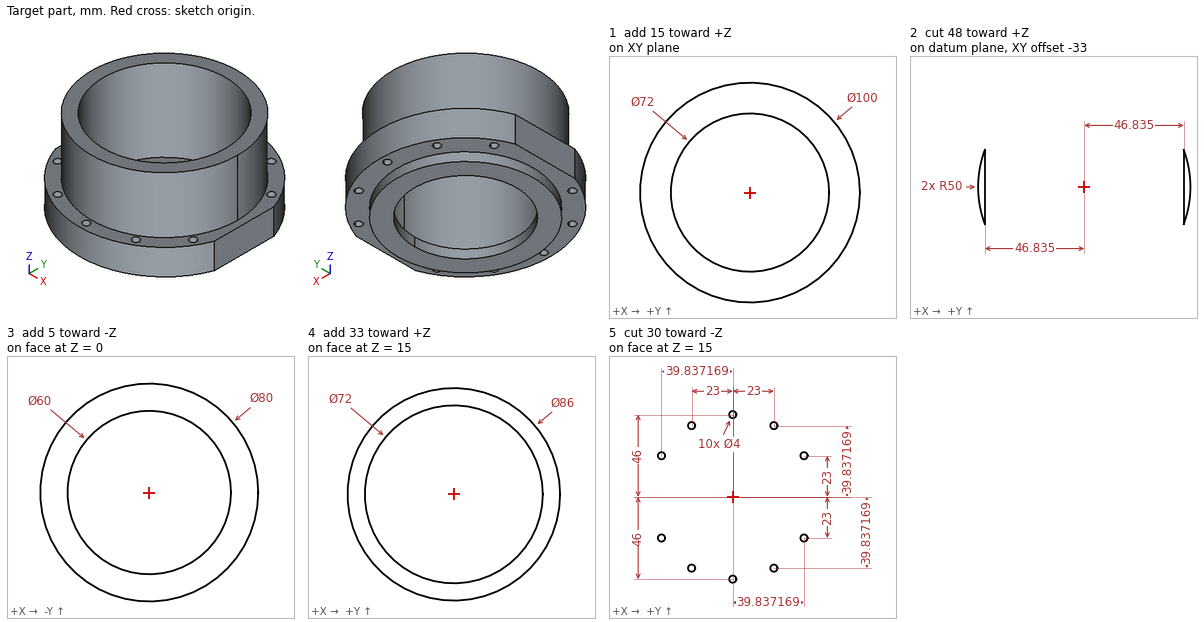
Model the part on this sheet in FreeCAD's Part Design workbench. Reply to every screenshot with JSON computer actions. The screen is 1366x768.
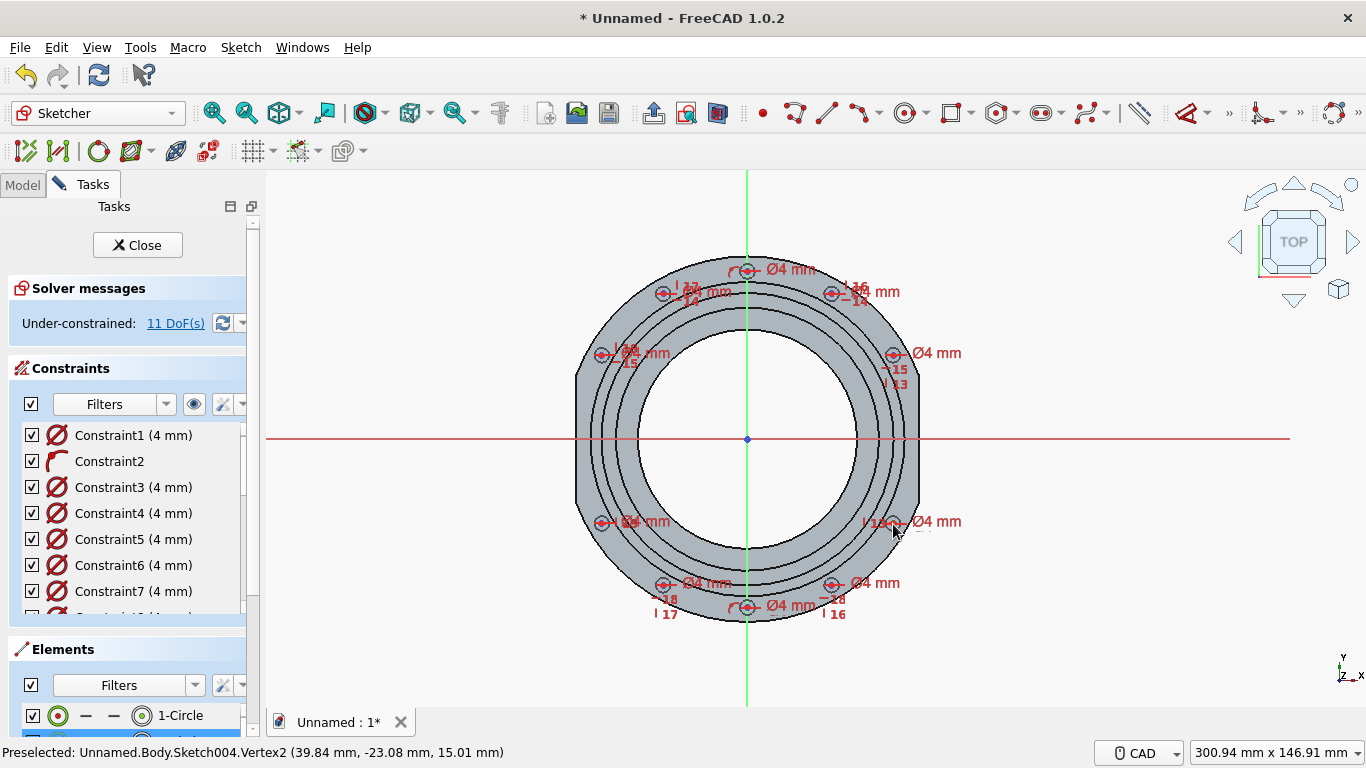
{"action": "left_click", "coordinate": [602, 523]}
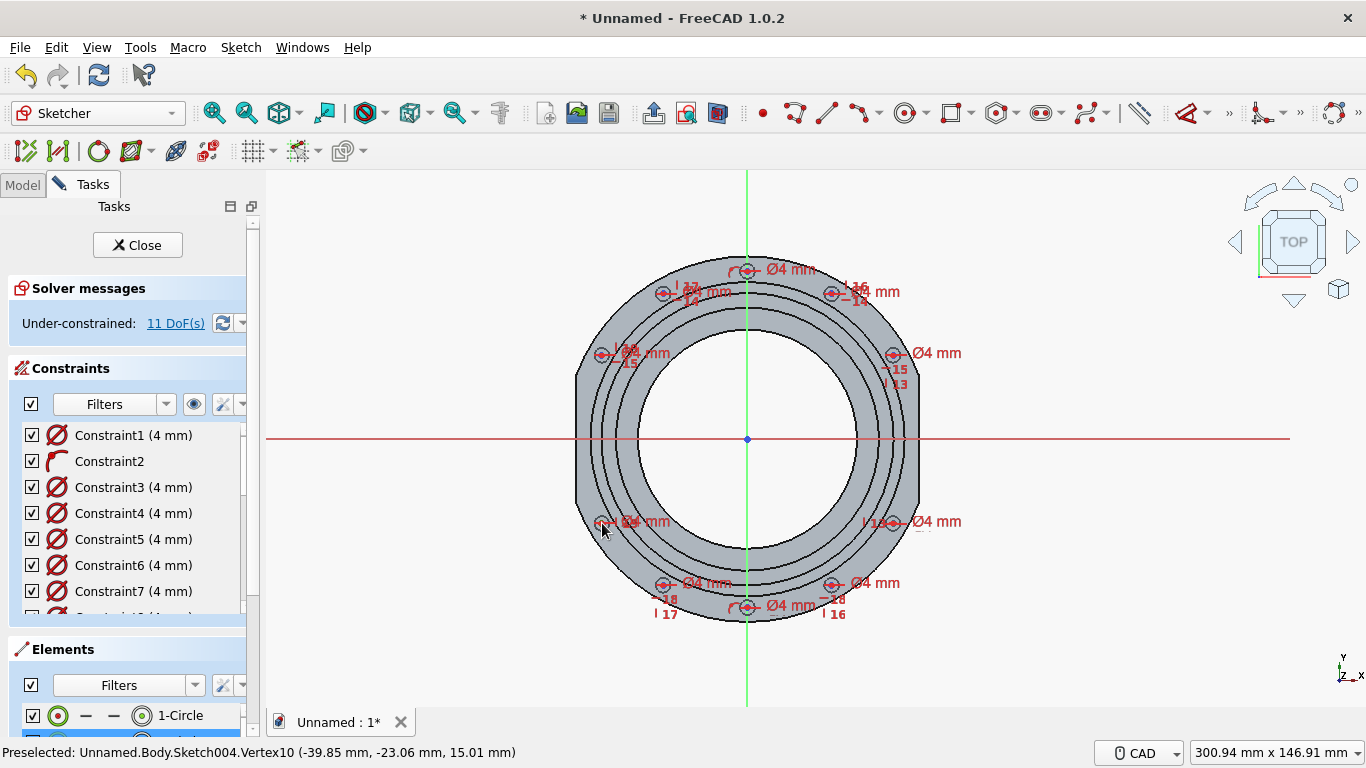
{"action": "key", "text": "h"}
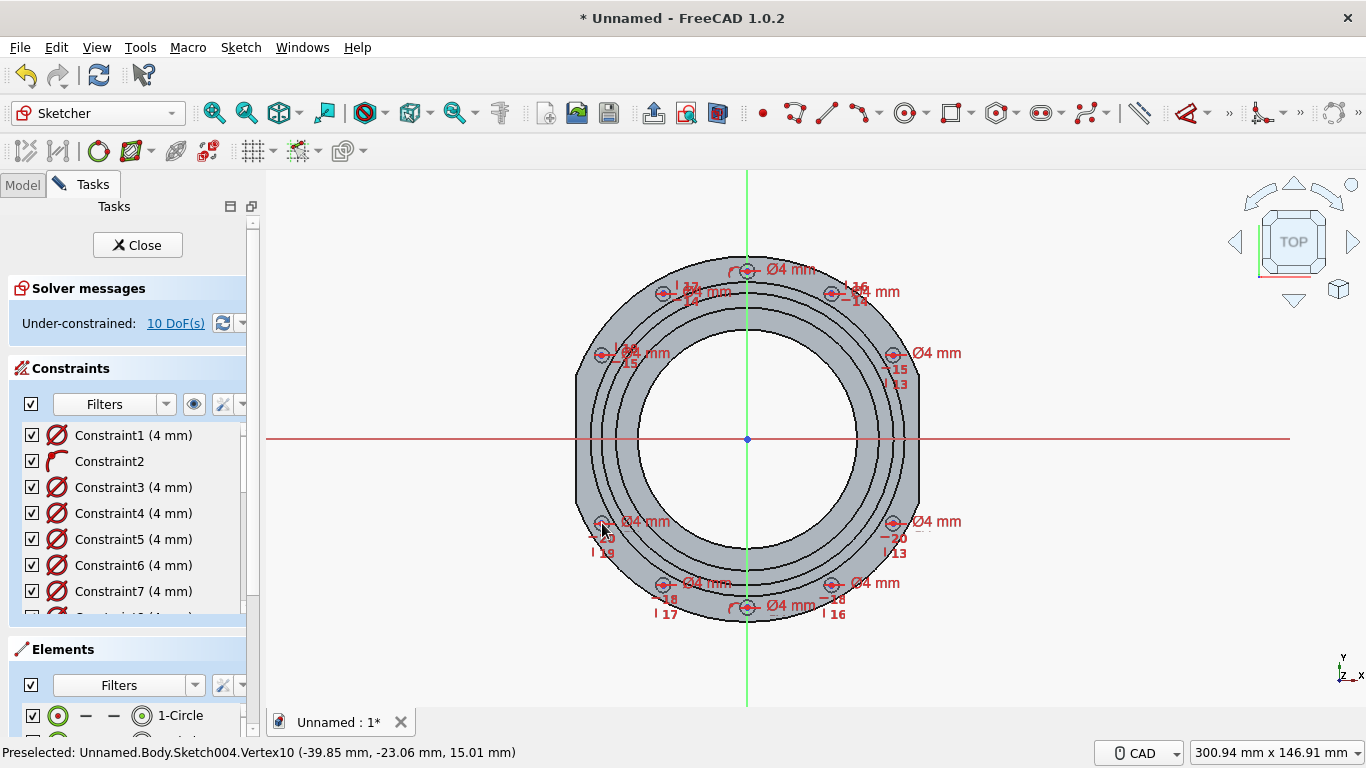
{"action": "left_click", "coordinate": [1186, 114]}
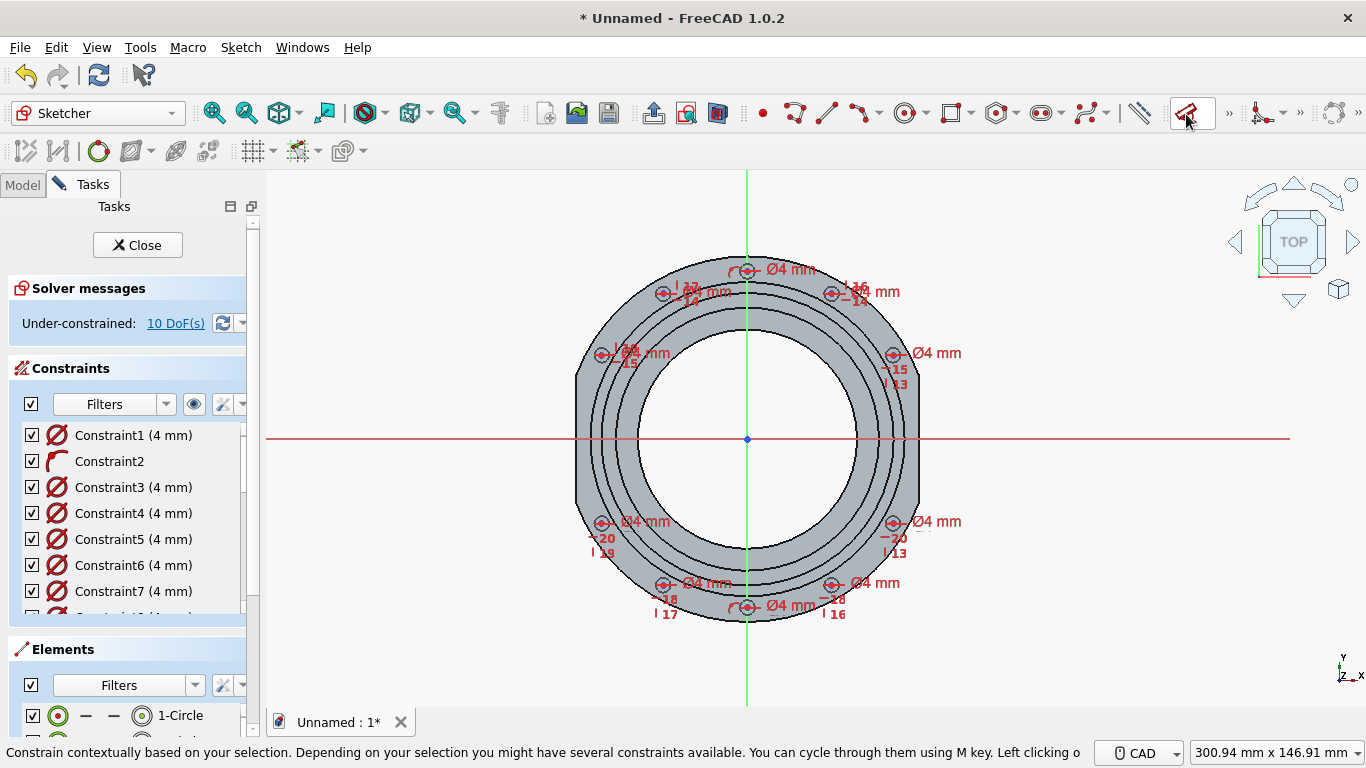
{"action": "left_click", "coordinate": [747, 271]}
{"action": "left_click", "coordinate": [781, 355]}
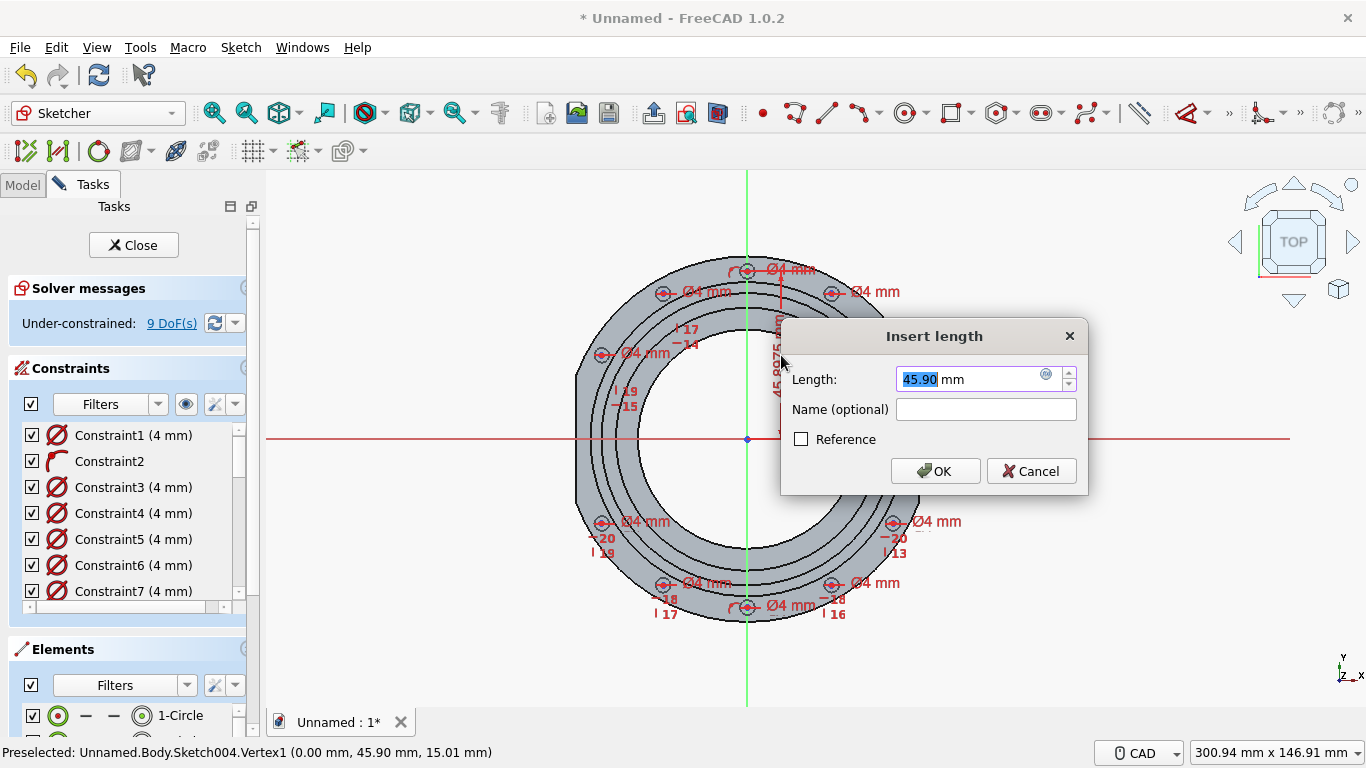
{"action": "type", "text": "46"}
{"action": "key", "text": "Return"}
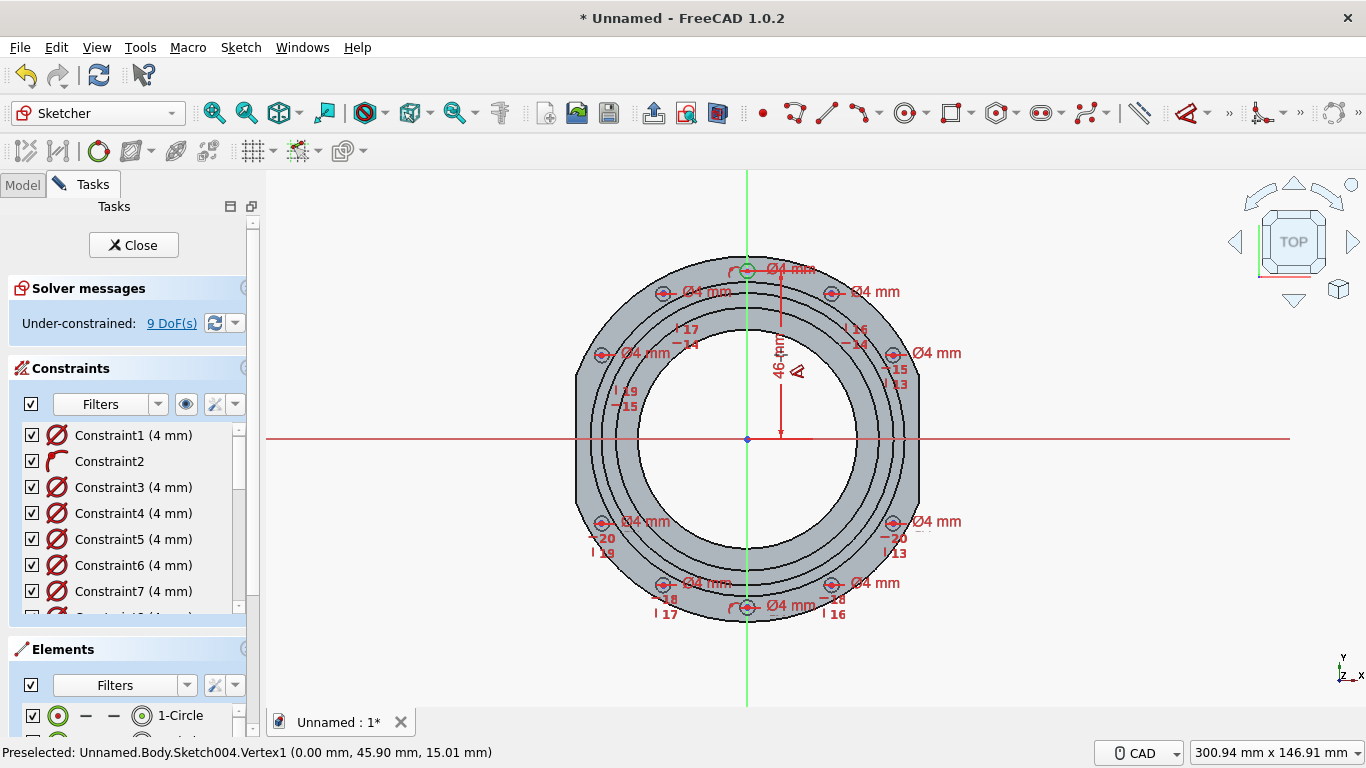
{"action": "left_click", "coordinate": [893, 524]}
{"action": "left_click", "coordinate": [927, 481]}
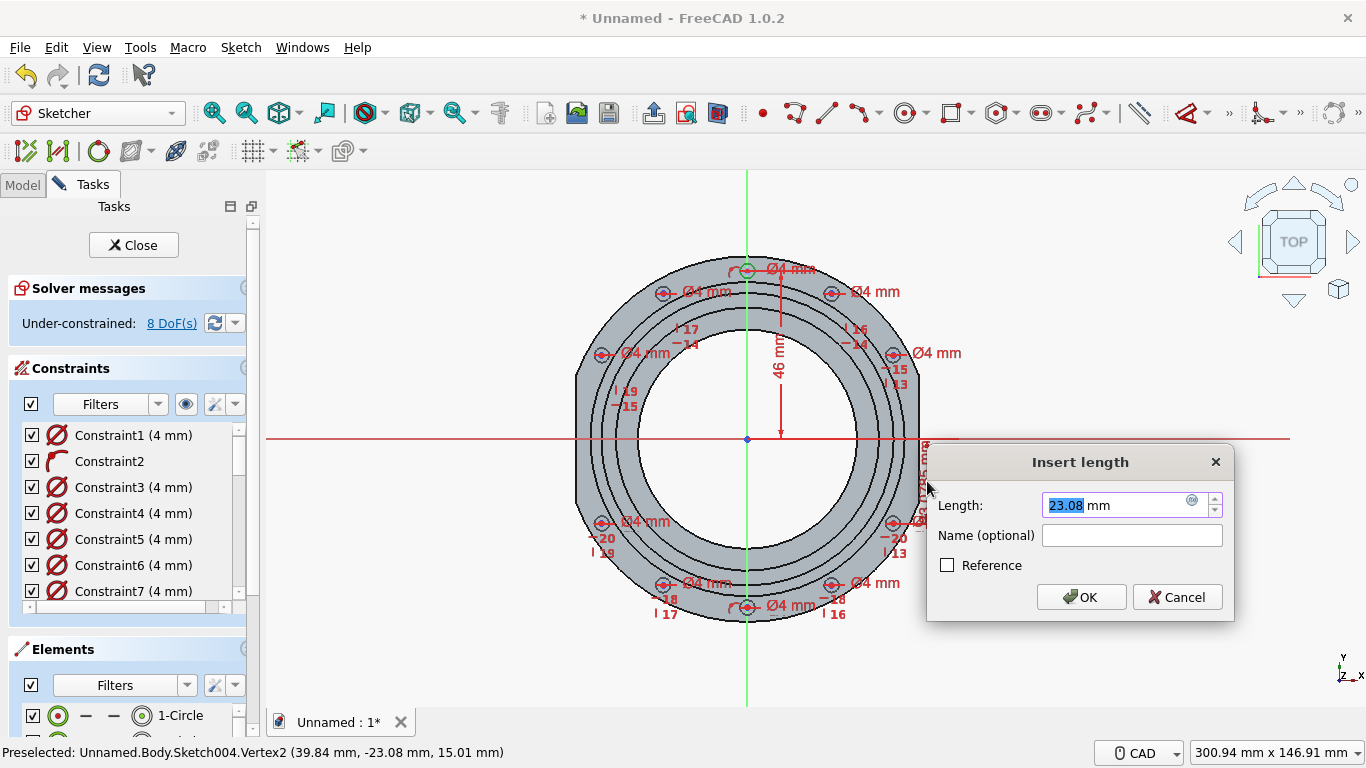
{"action": "type", "text": "23"}
{"action": "key", "text": "Return"}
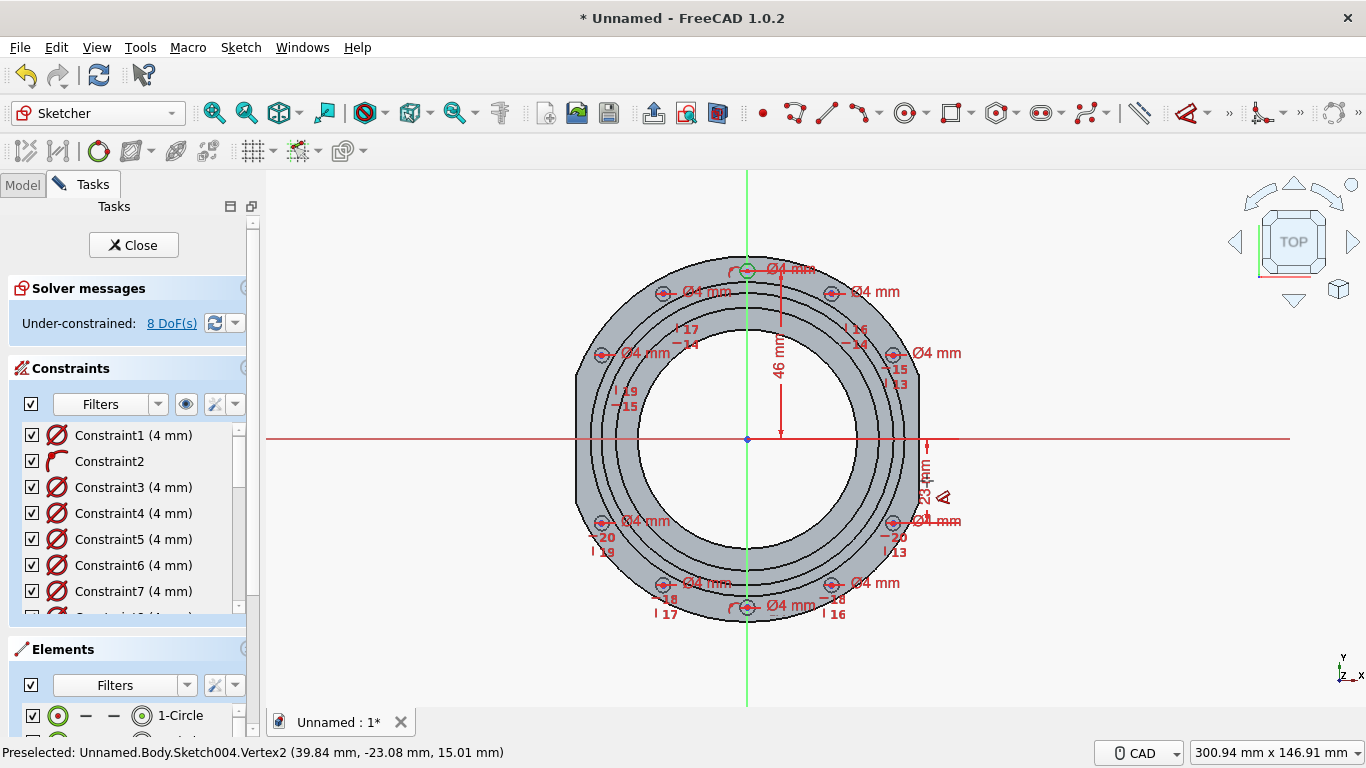
{"action": "left_click", "coordinate": [832, 294]}
{"action": "left_click", "coordinate": [790, 260]}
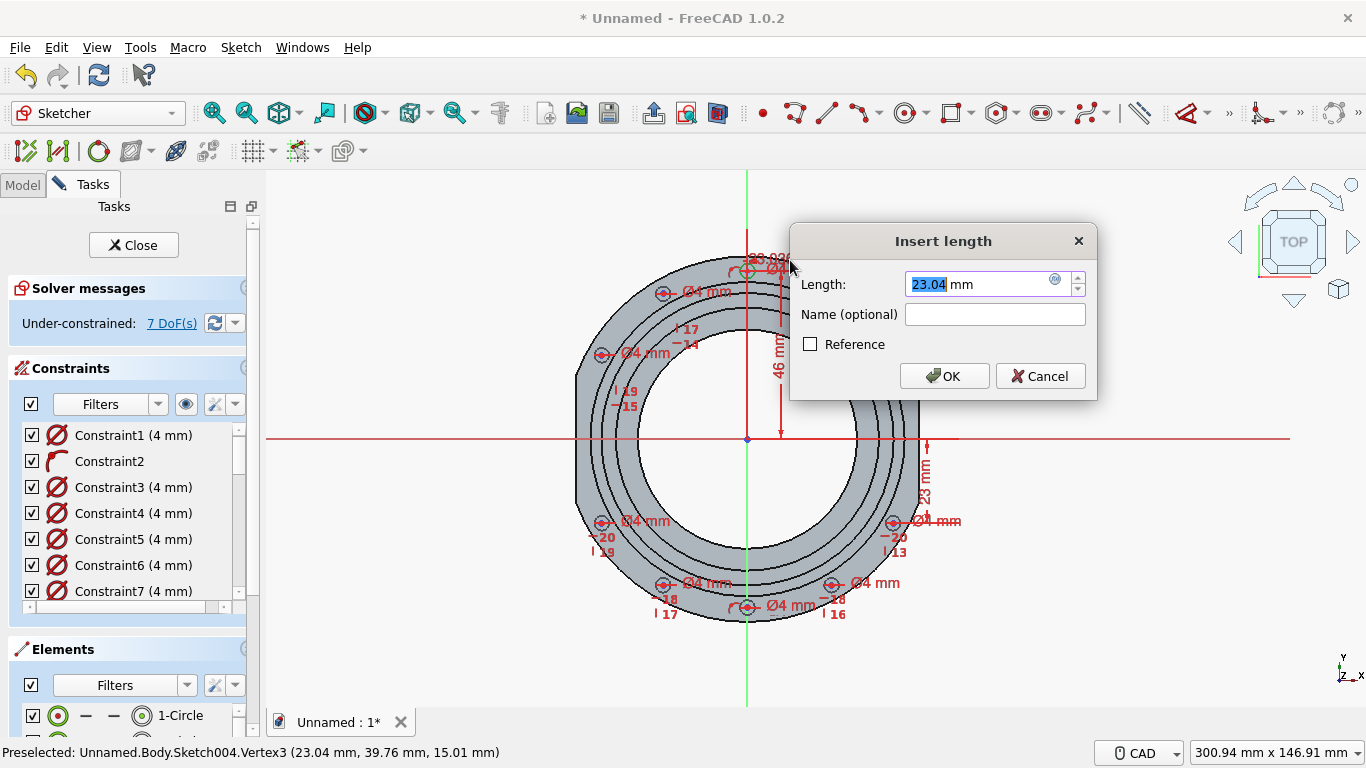
{"action": "type", "text": "23"}
{"action": "key", "text": "Return"}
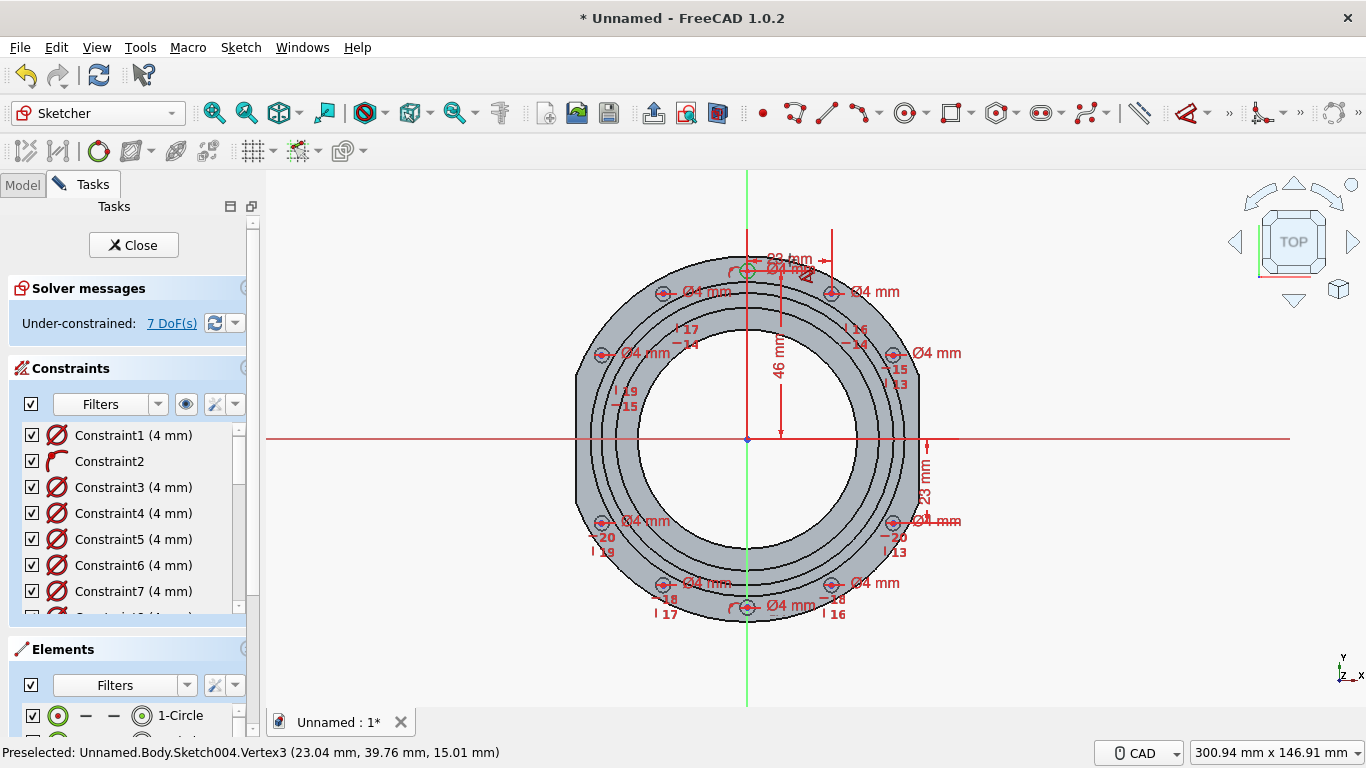
{"action": "left_click", "coordinate": [893, 355]}
{"action": "left_click", "coordinate": [927, 397]}